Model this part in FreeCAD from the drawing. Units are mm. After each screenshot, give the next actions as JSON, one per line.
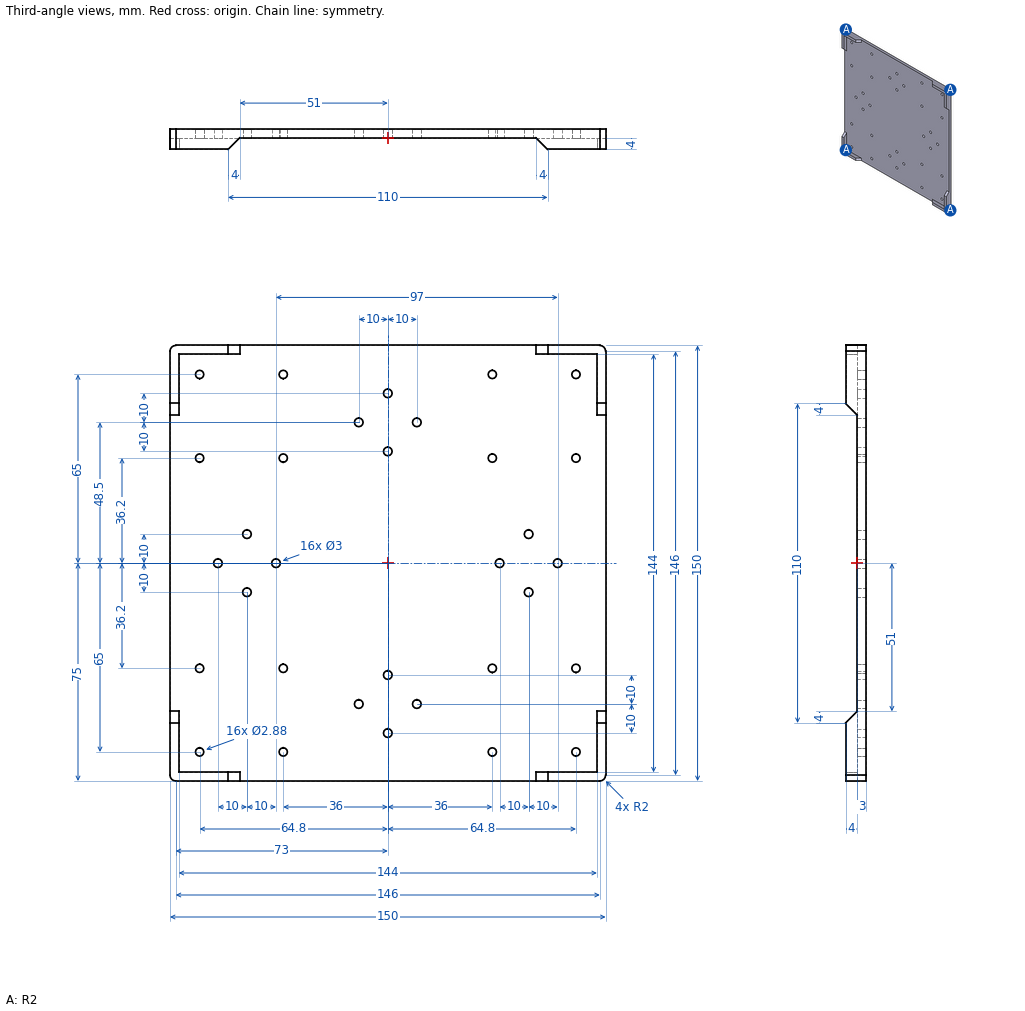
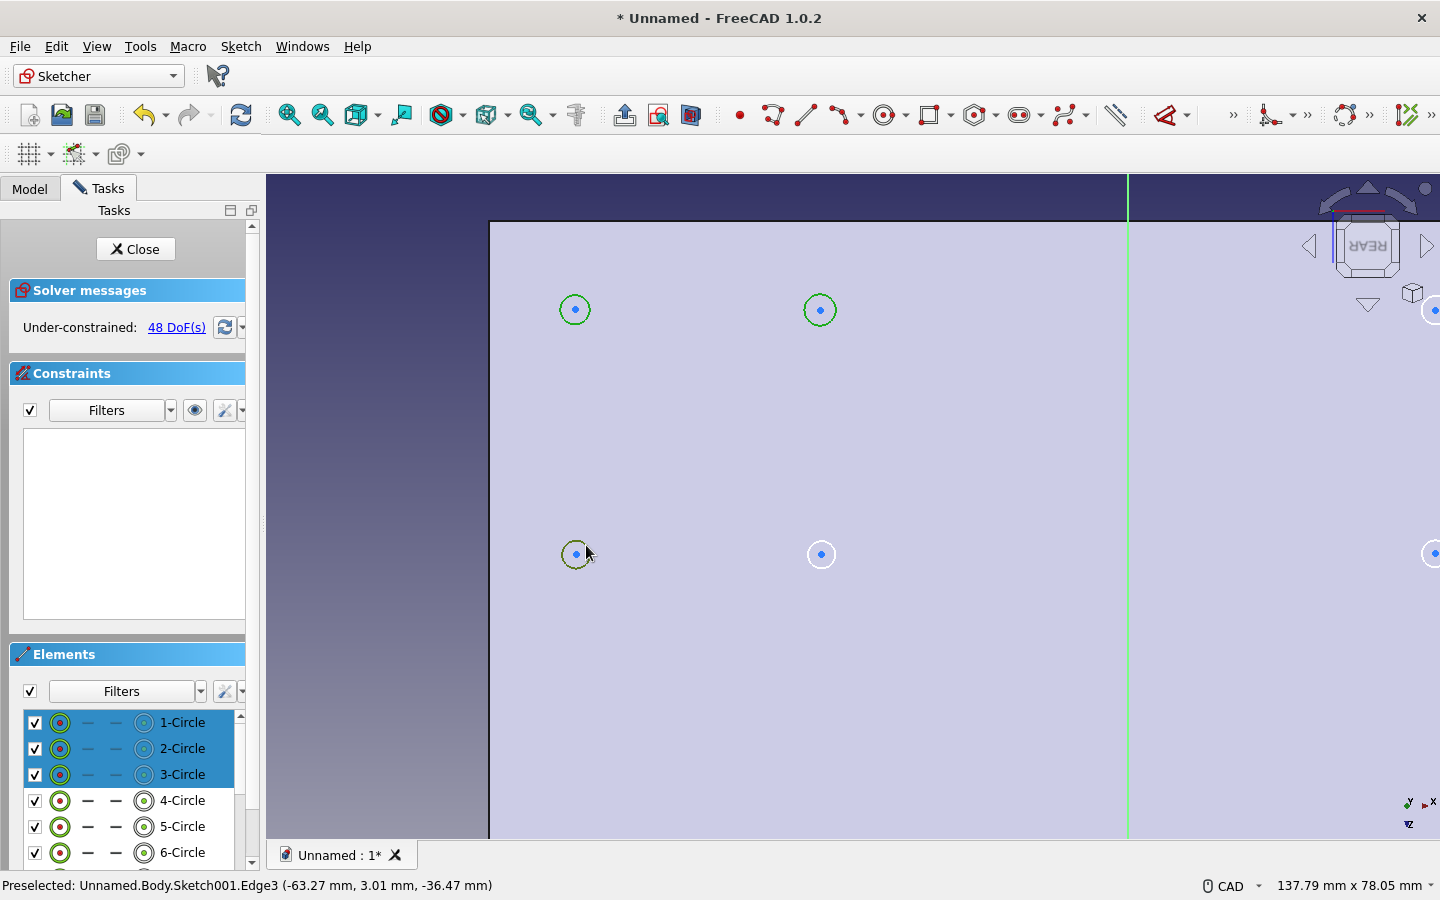
{"action": "left_click", "coordinate": [831, 545]}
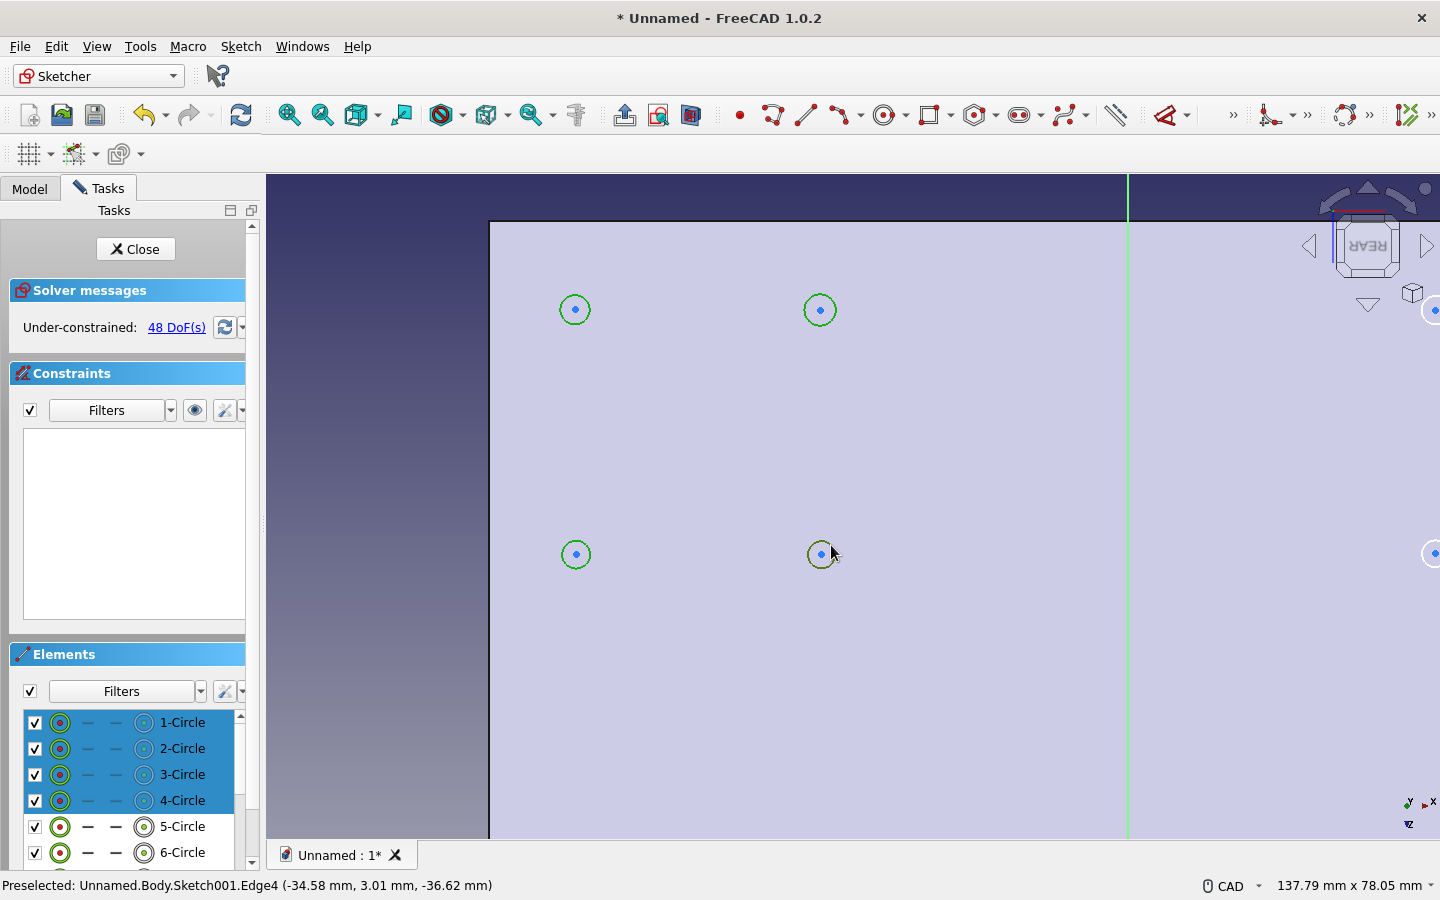
{"action": "scroll", "coordinate": [584, 301], "scroll_direction": "down", "scroll_amount": 5}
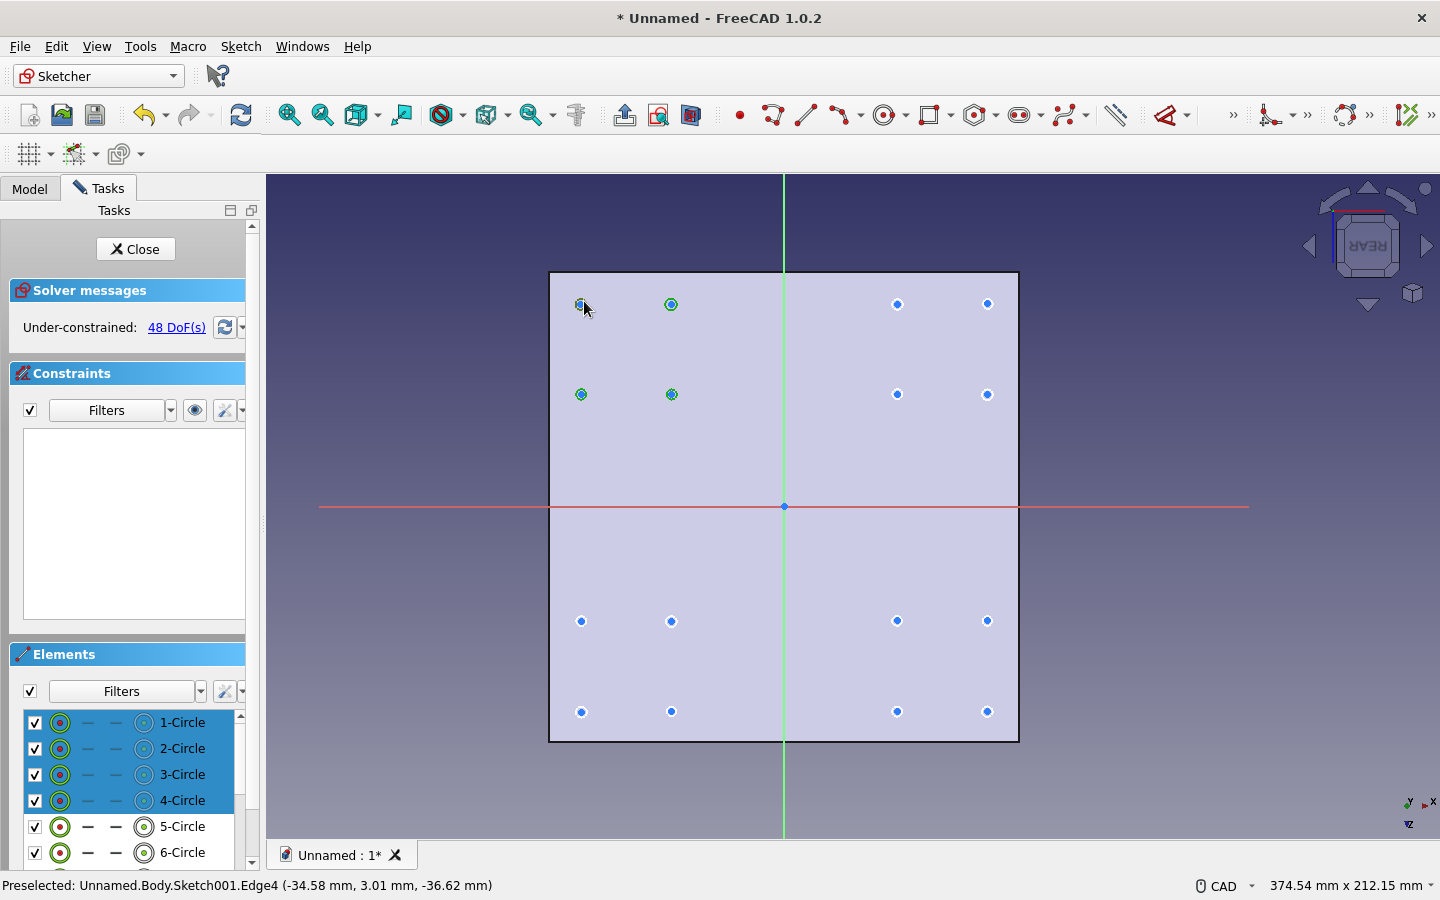
{"action": "scroll", "coordinate": [901, 301], "scroll_direction": "up", "scroll_amount": 5}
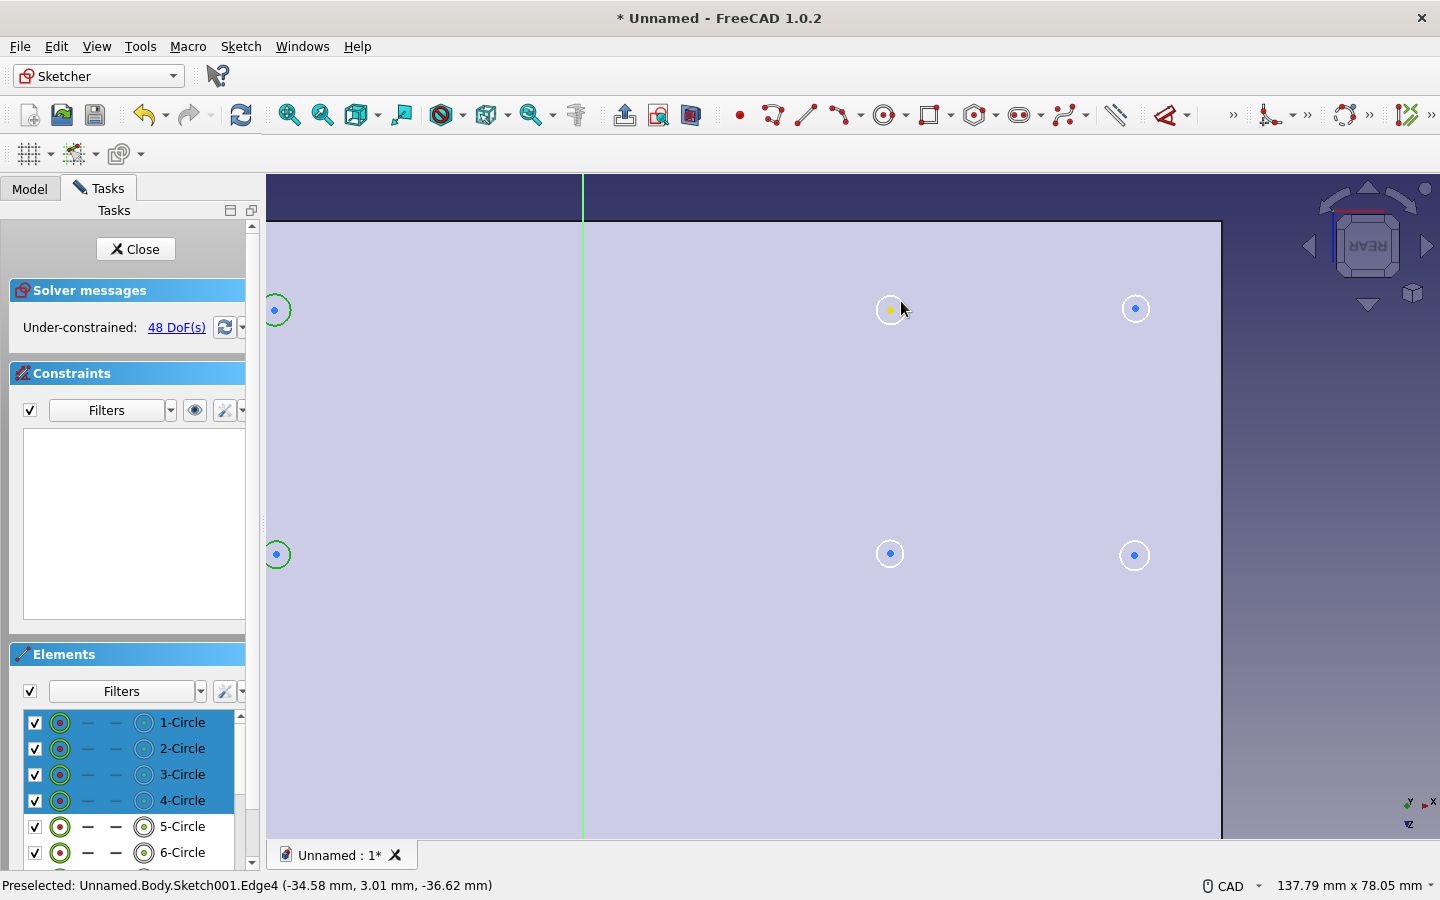
{"action": "left_click", "coordinate": [901, 300]}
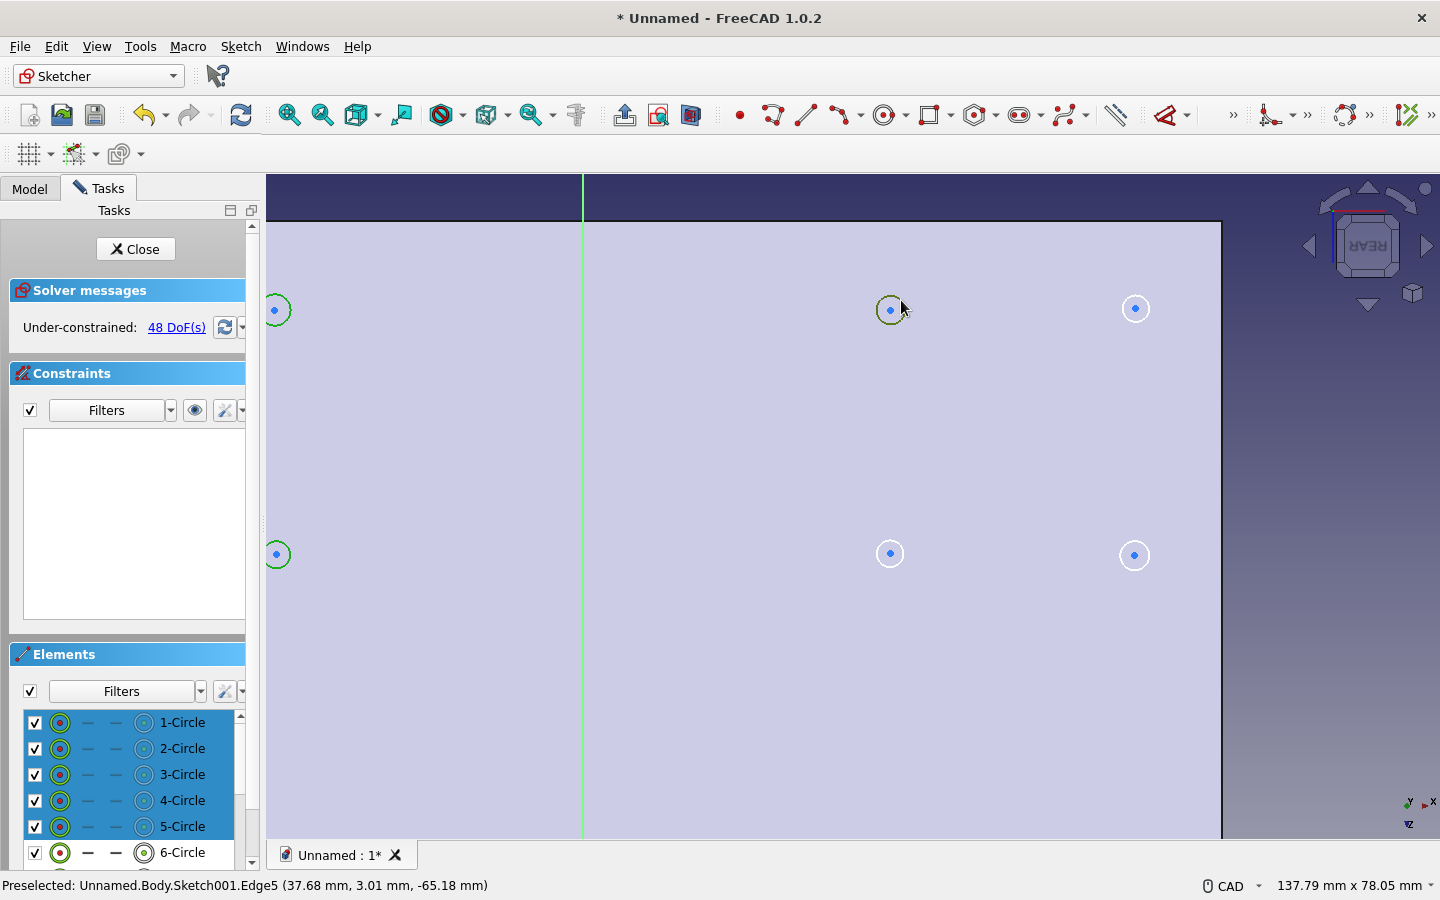
{"action": "left_click", "coordinate": [1145, 299]}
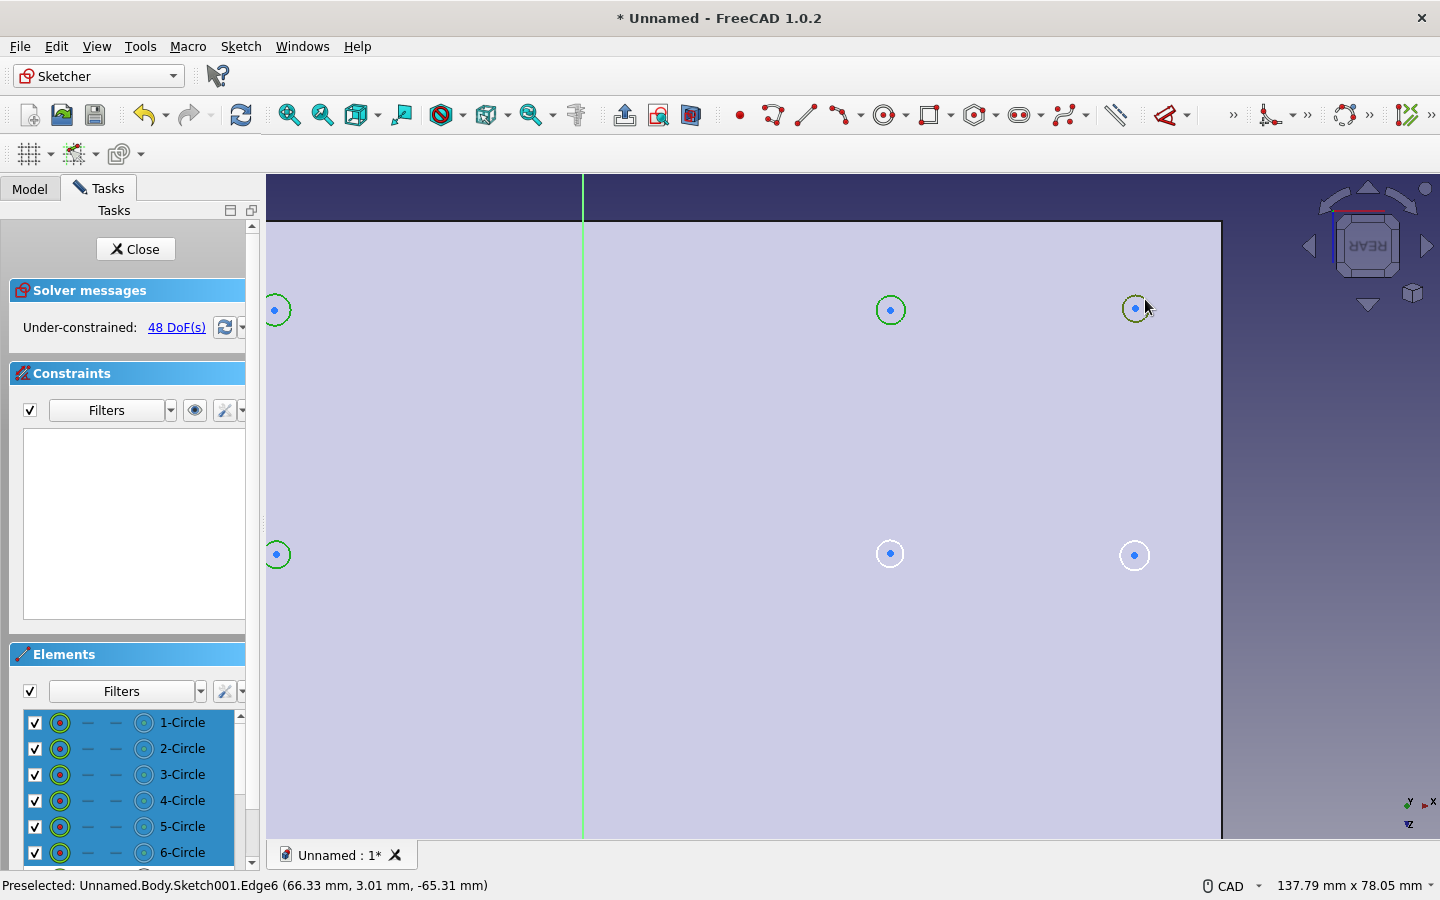
{"action": "left_click", "coordinate": [1145, 545]}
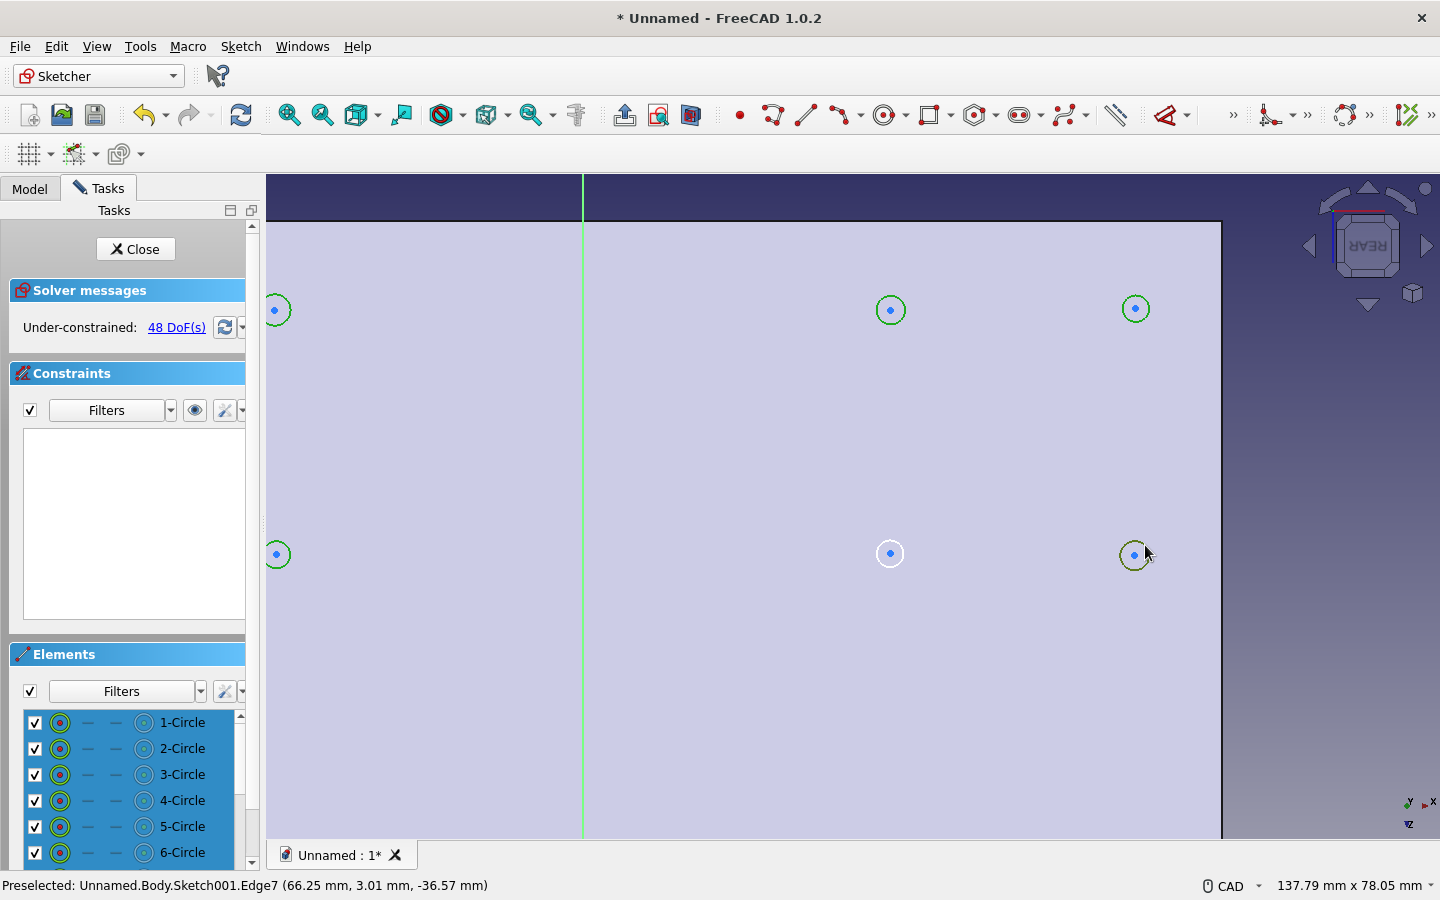
{"action": "left_click", "coordinate": [900, 544]}